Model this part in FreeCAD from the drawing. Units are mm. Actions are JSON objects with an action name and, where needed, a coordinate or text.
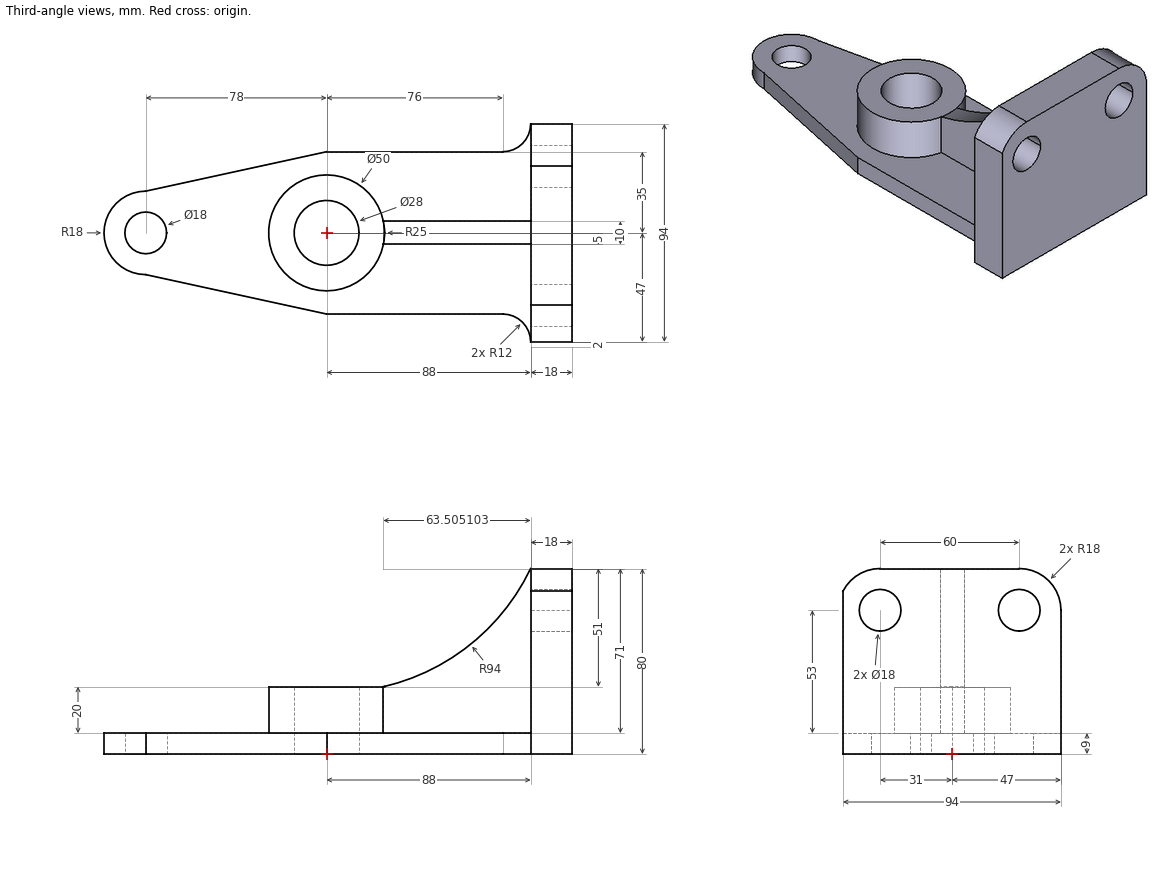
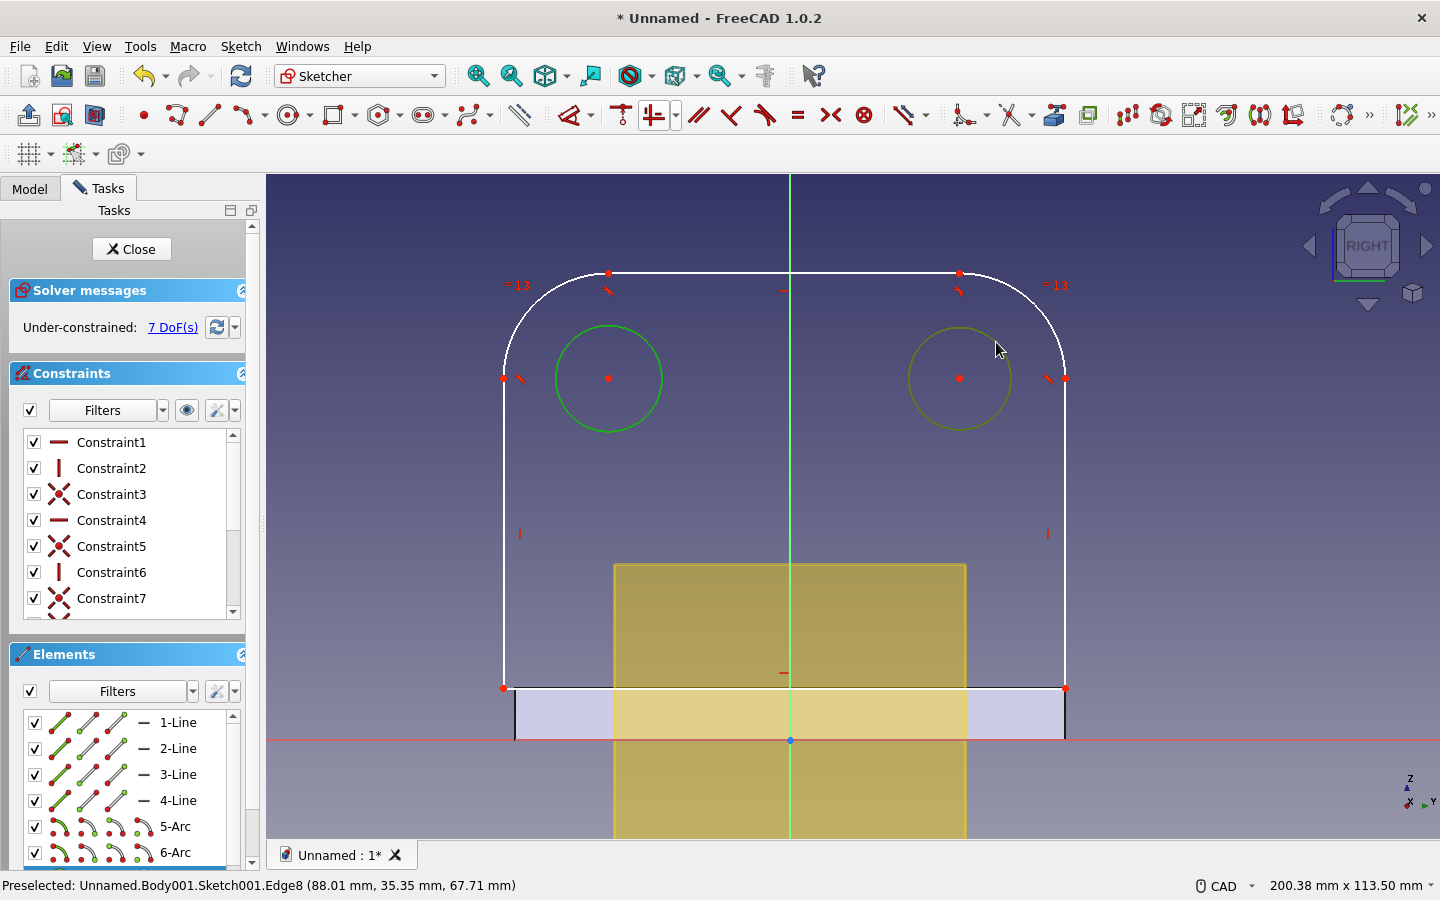
{"action": "key", "text": "e"}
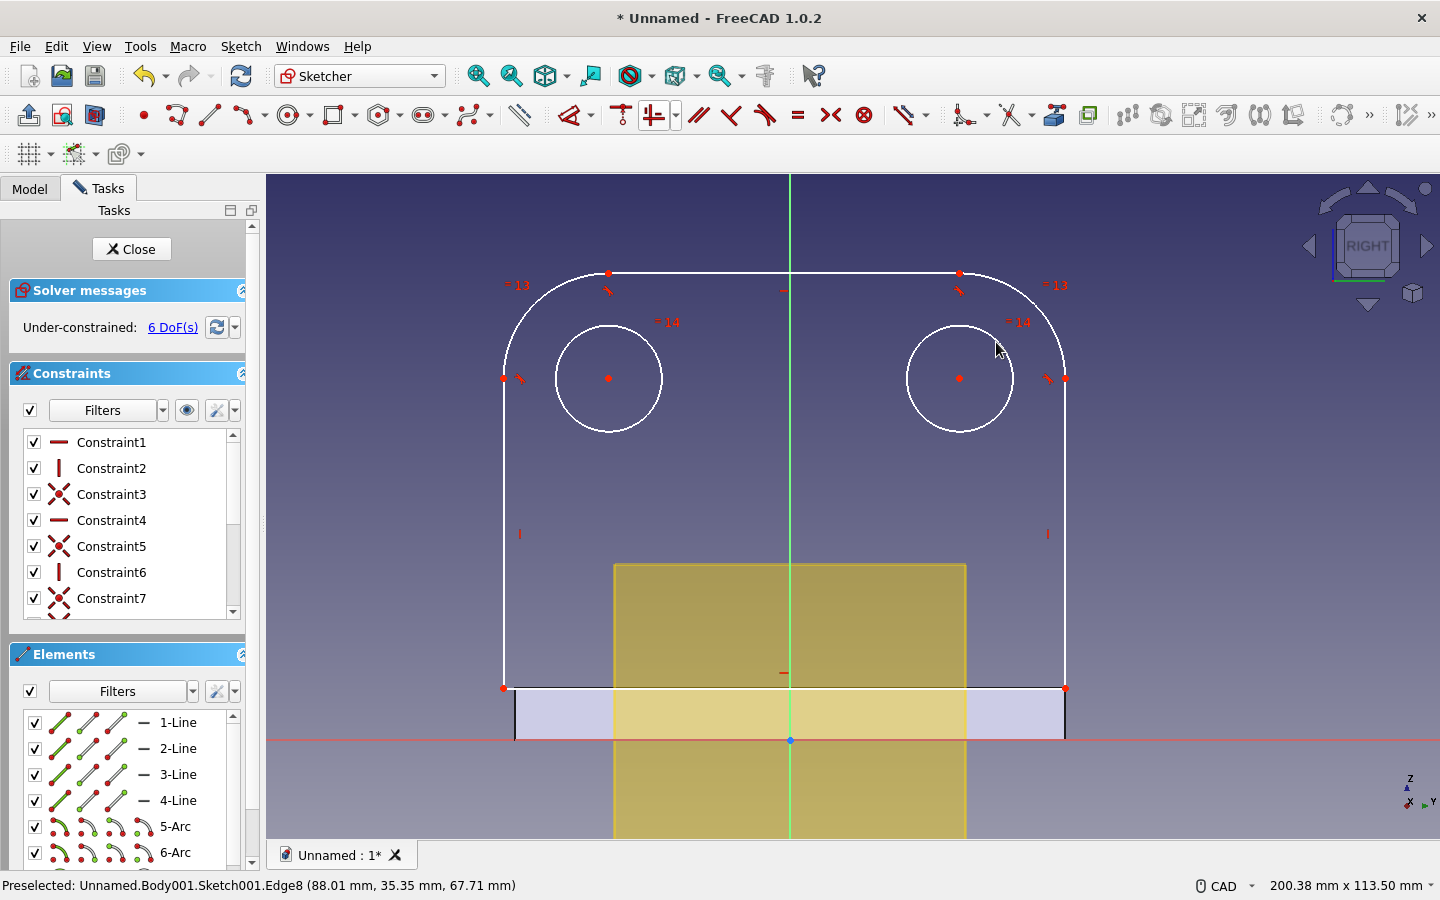
{"action": "key", "text": "d"}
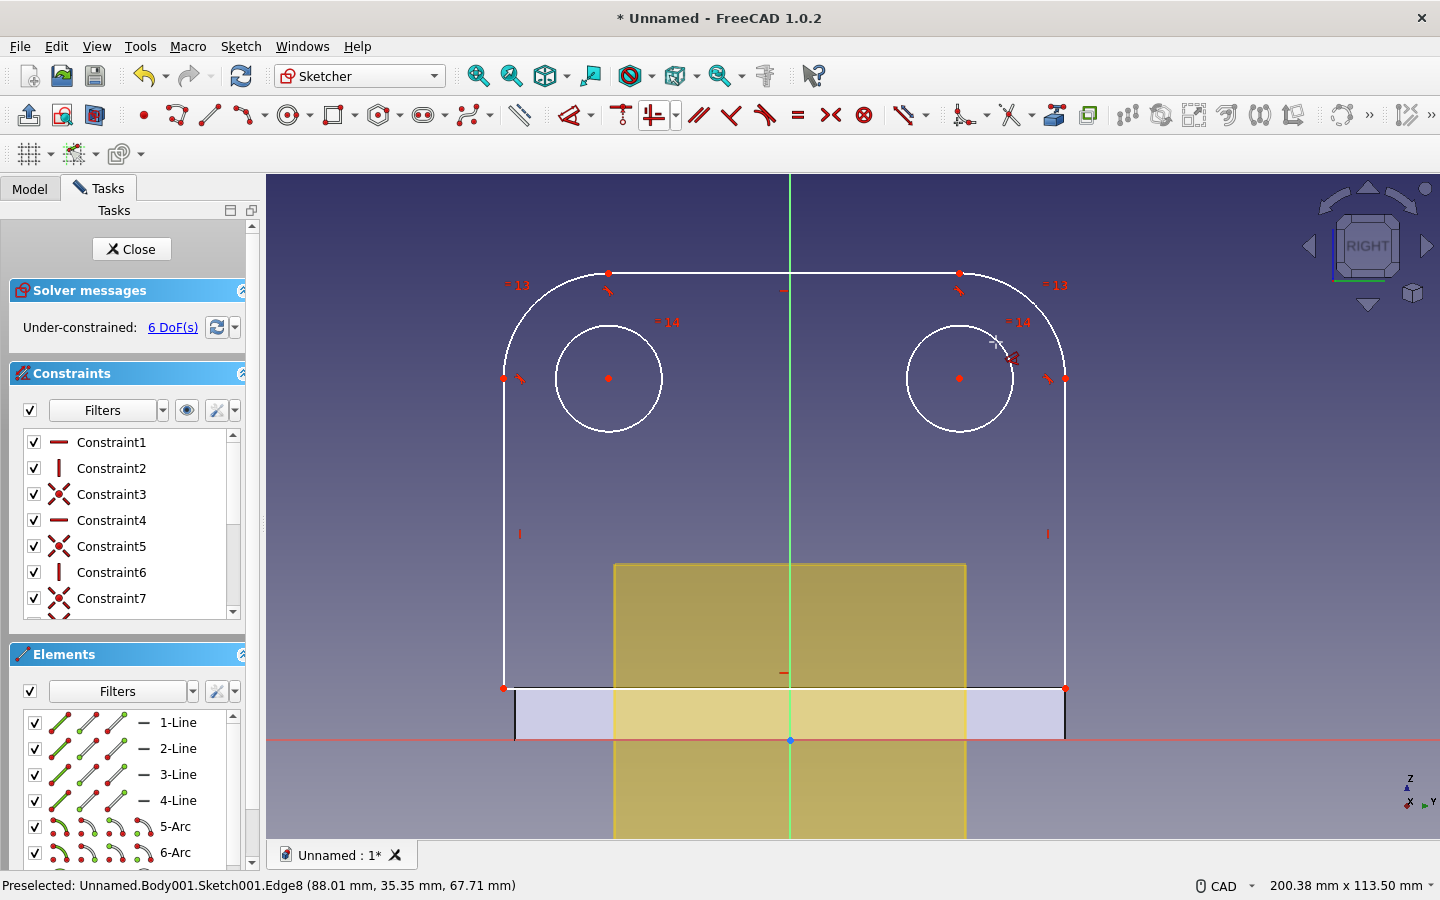
{"action": "left_click", "coordinate": [561, 285]}
{"action": "left_click", "coordinate": [546, 257]}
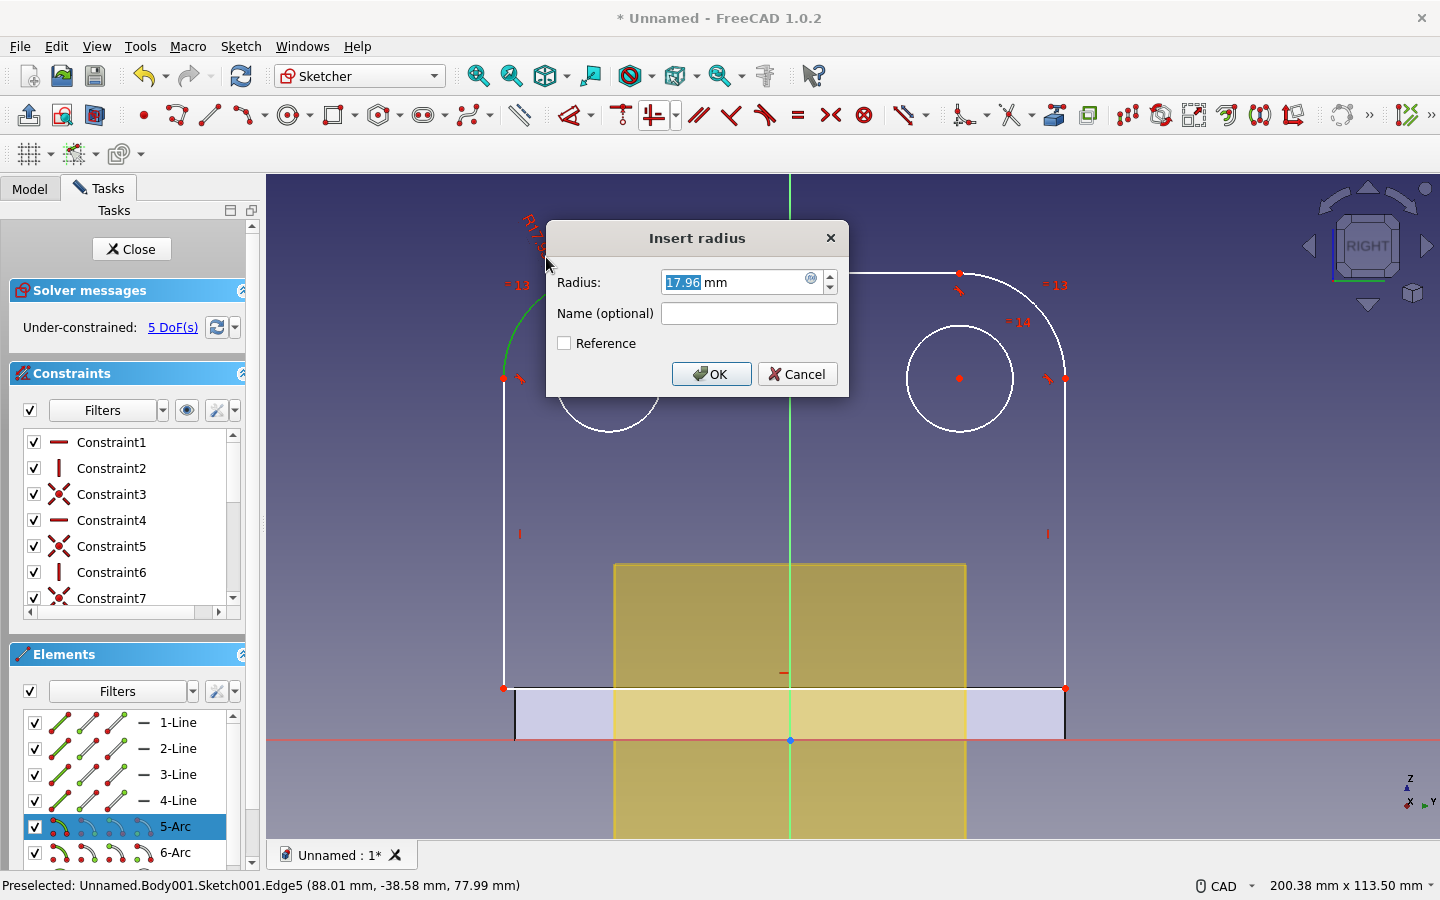
{"action": "type", "text": "18"}
{"action": "key", "text": "Return"}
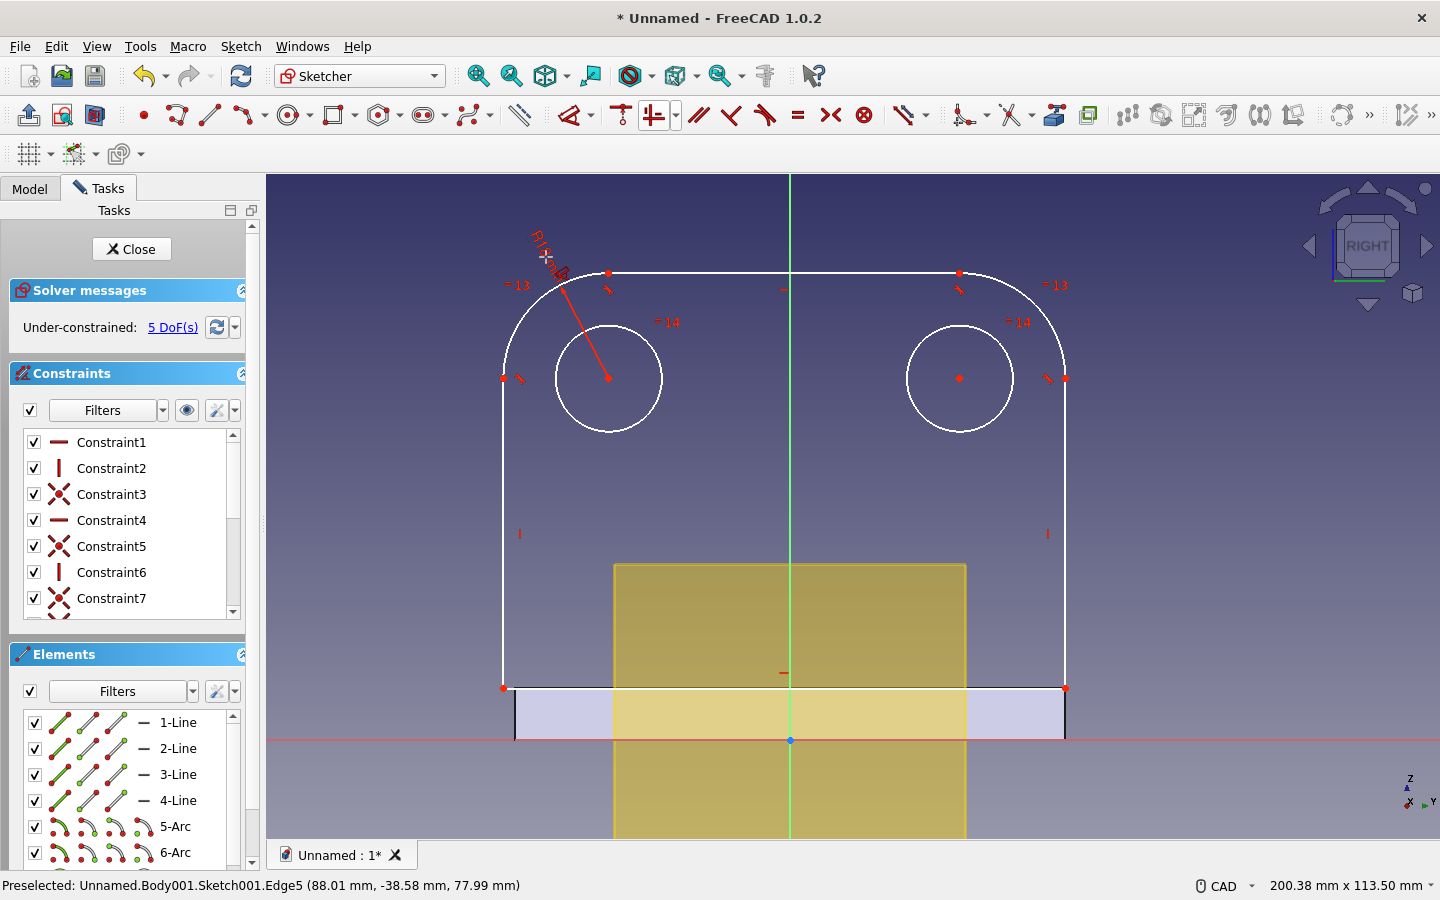
{"action": "left_click", "coordinate": [646, 341]}
{"action": "left_click", "coordinate": [668, 318]}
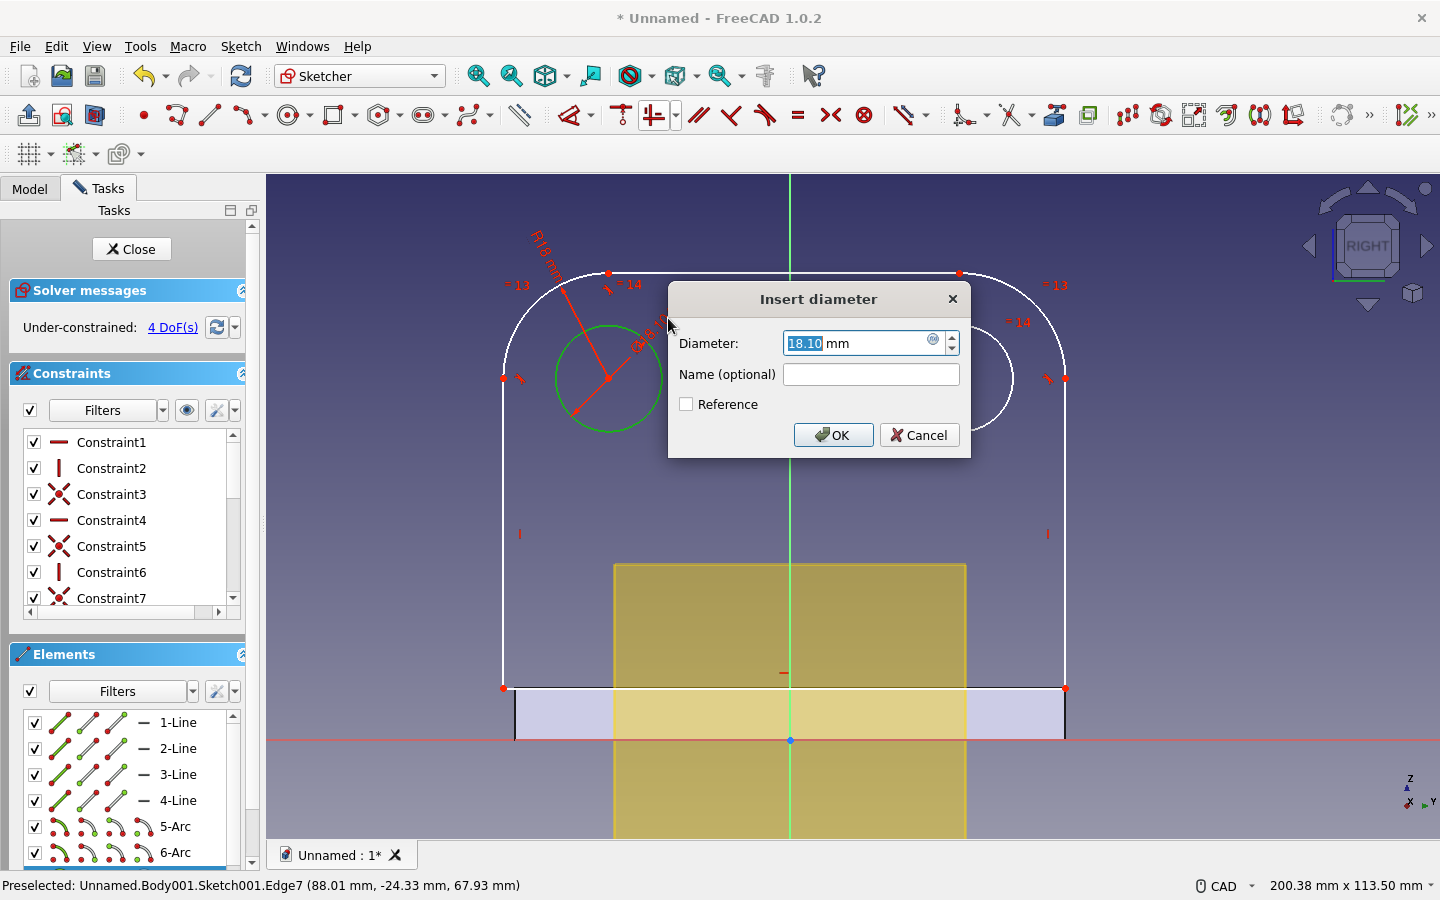
{"action": "type", "text": "18"}
{"action": "key", "text": "Return"}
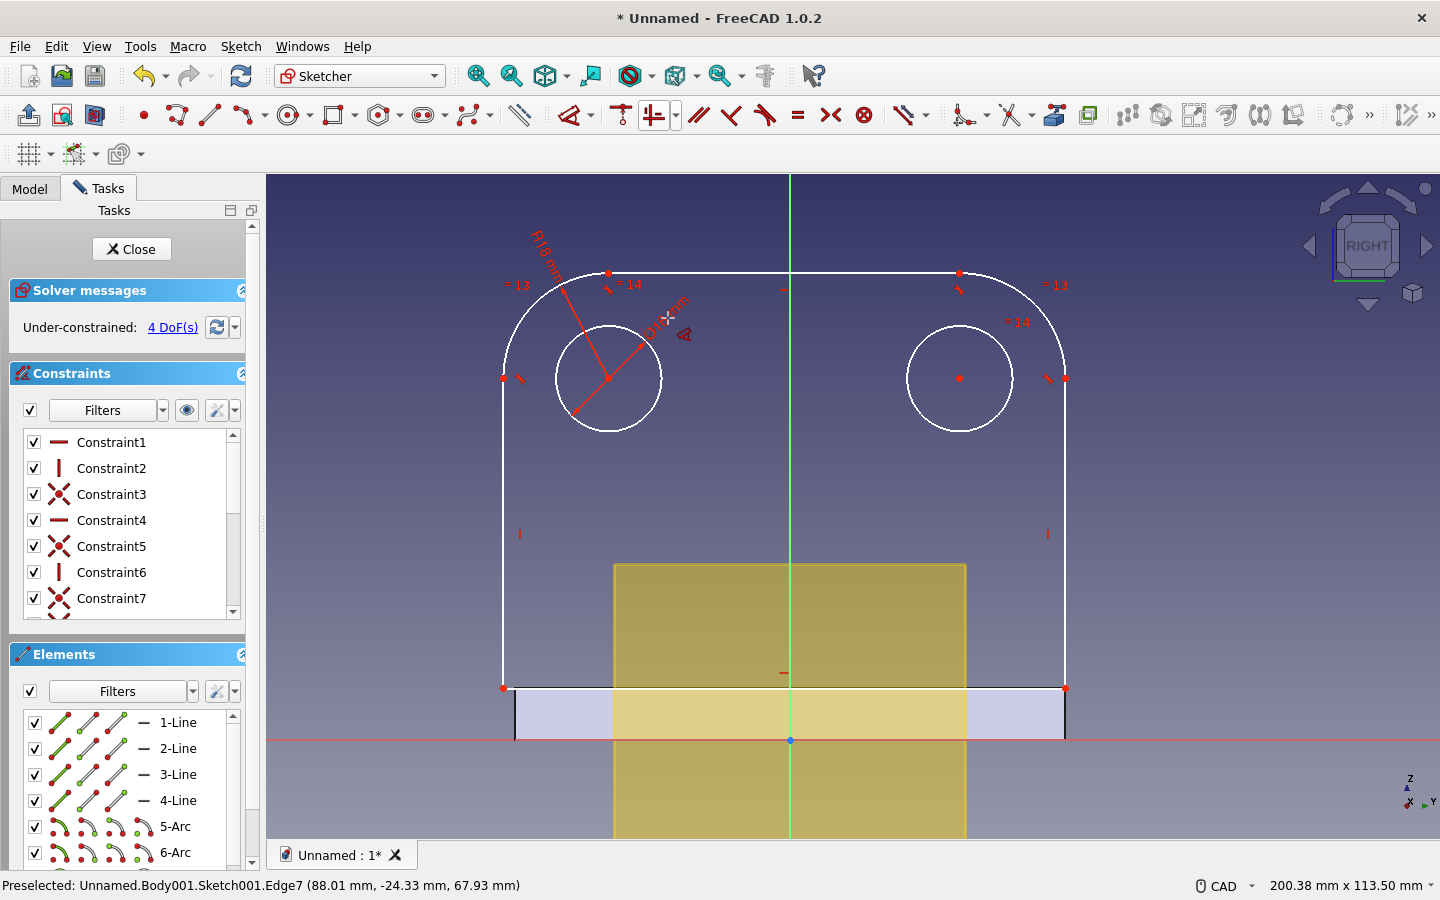
{"action": "left_click", "coordinate": [855, 273]}
{"action": "left_click", "coordinate": [704, 239]}